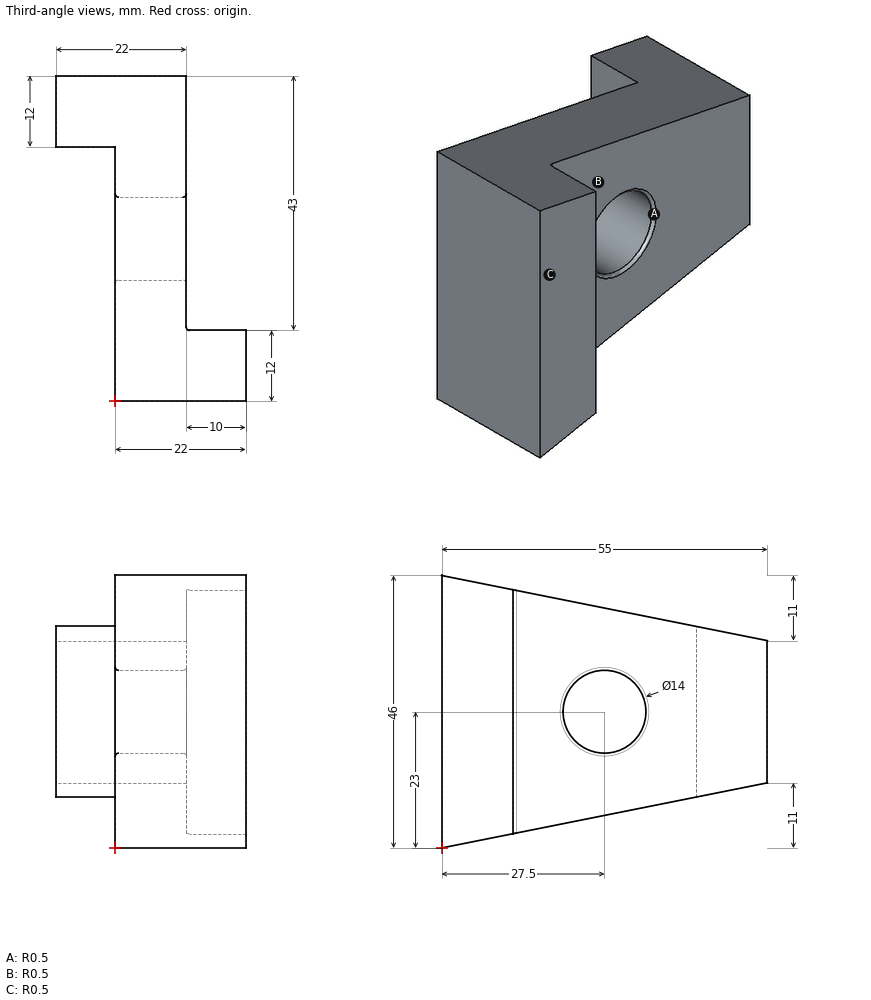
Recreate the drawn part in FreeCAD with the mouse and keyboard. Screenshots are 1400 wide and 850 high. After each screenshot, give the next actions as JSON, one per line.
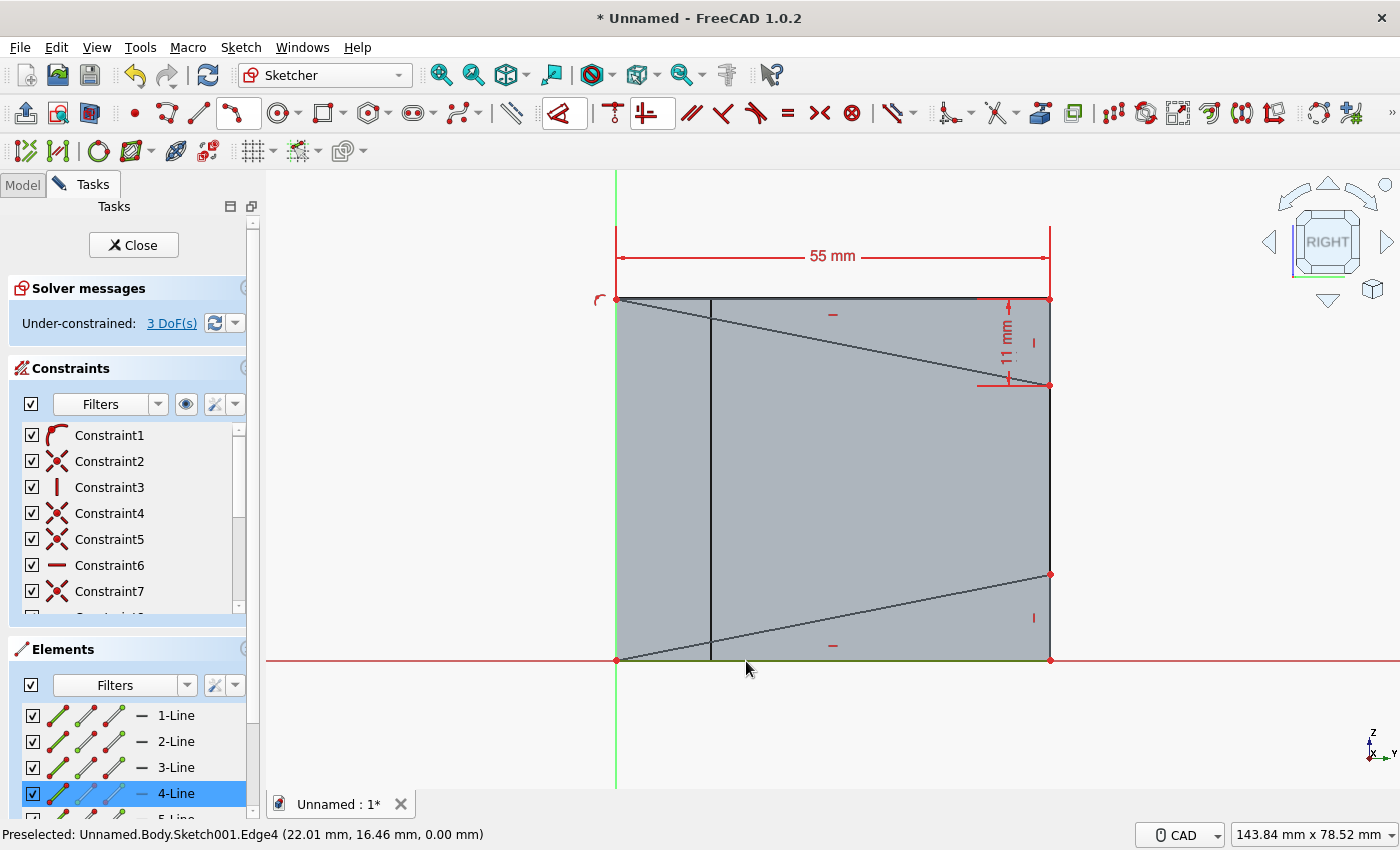
{"action": "key", "text": "l"}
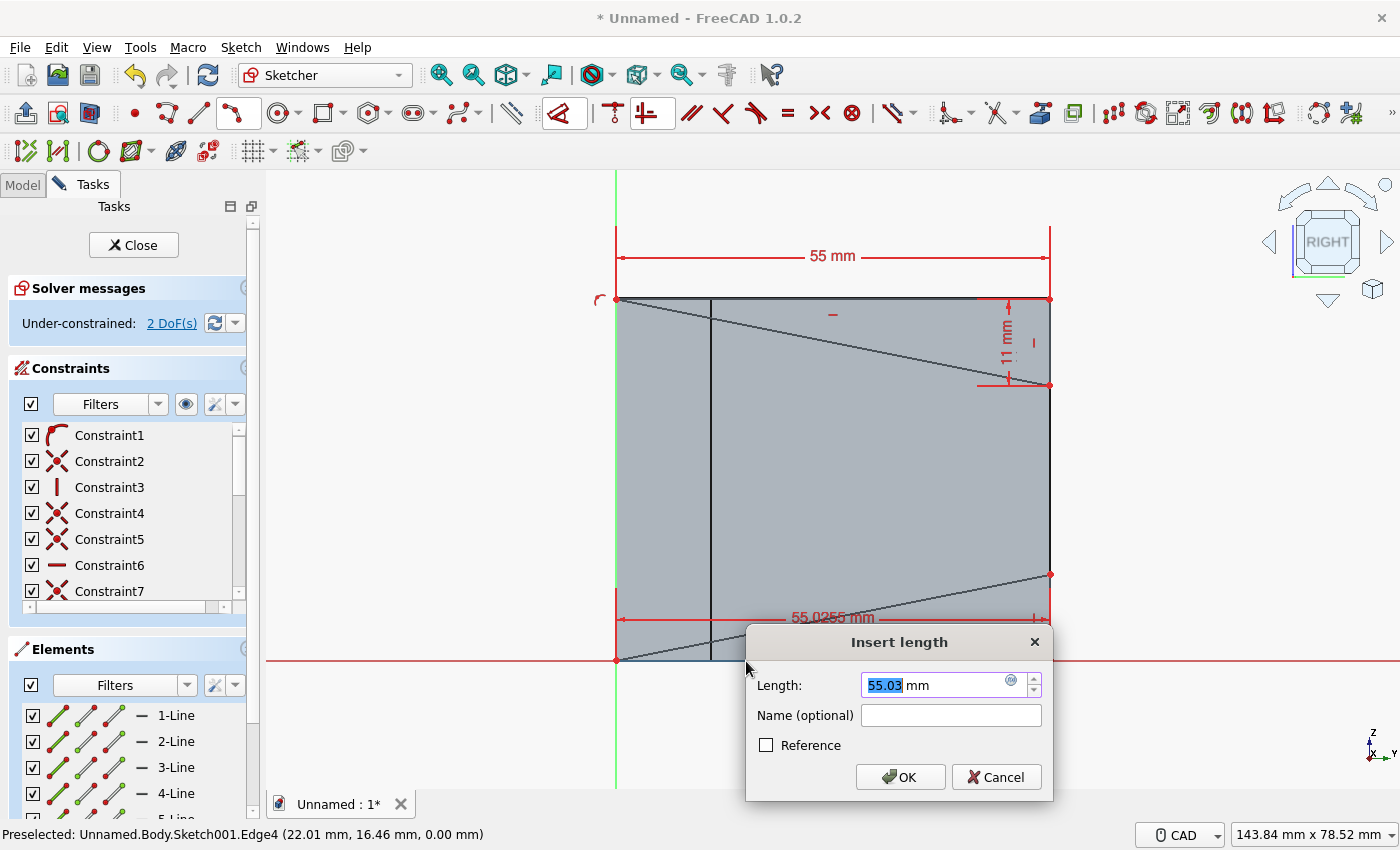
{"action": "type", "text": "55"}
{"action": "key", "text": "Return"}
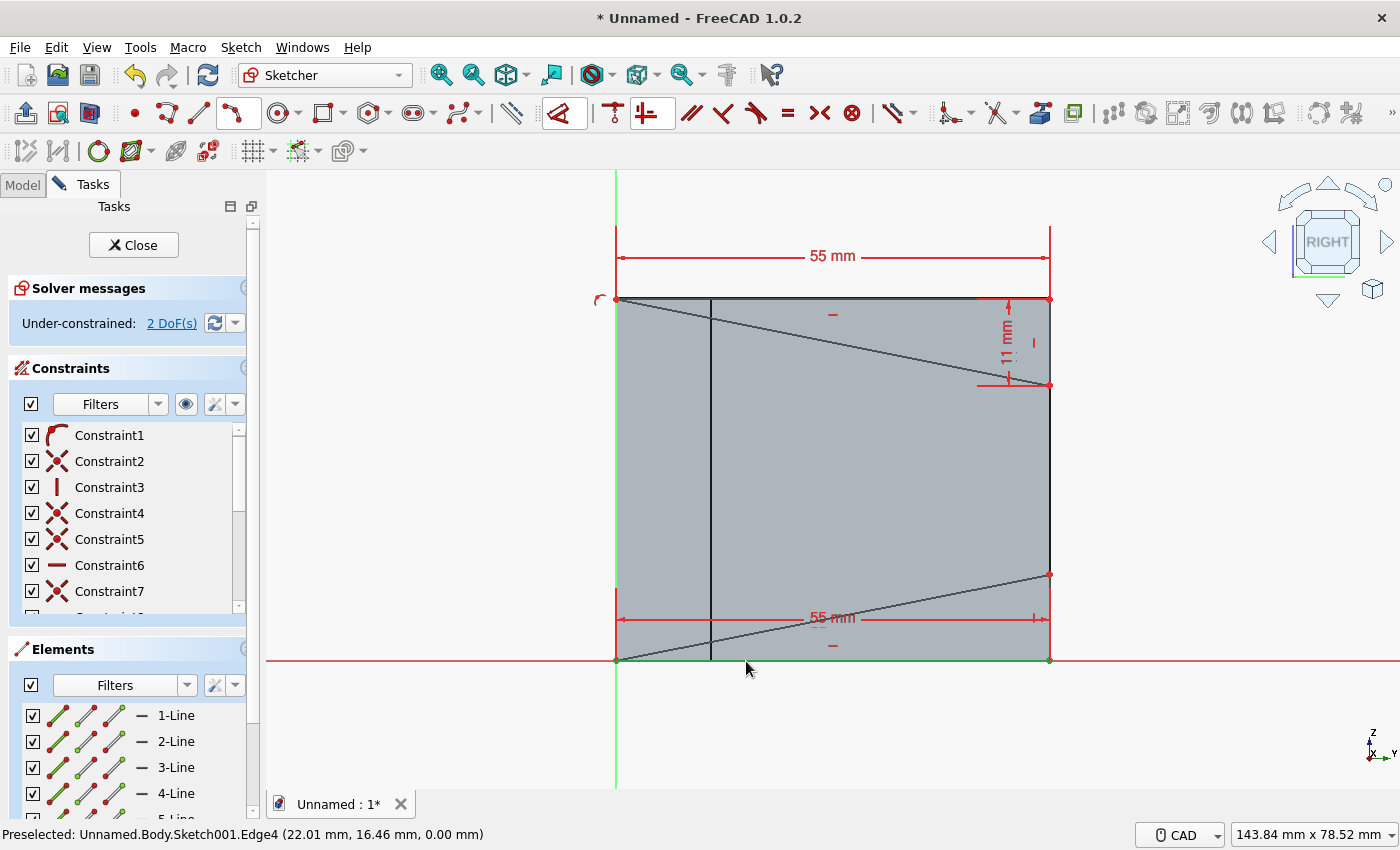
{"action": "left_click", "coordinate": [1050, 635]}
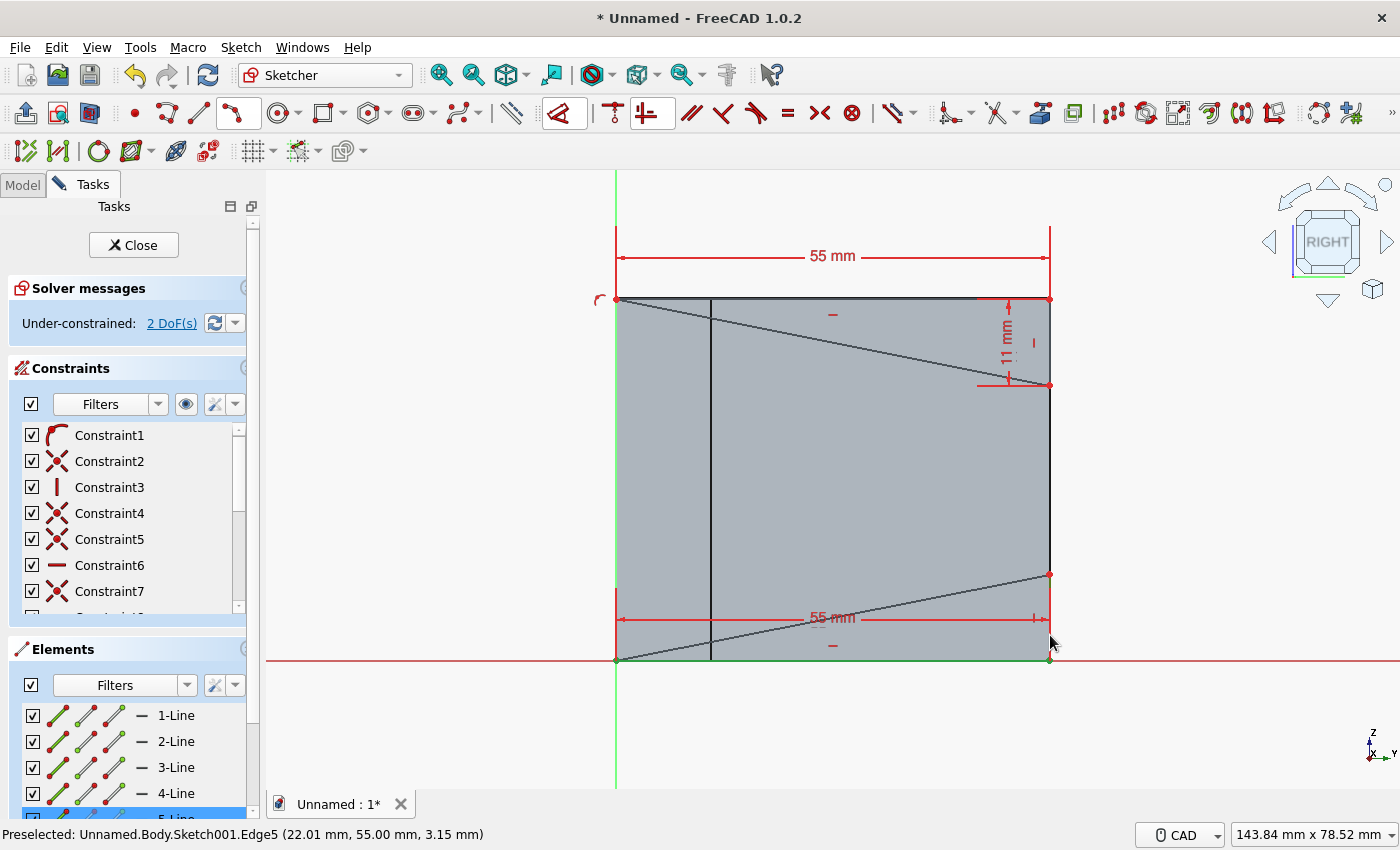
{"action": "key", "text": "i"}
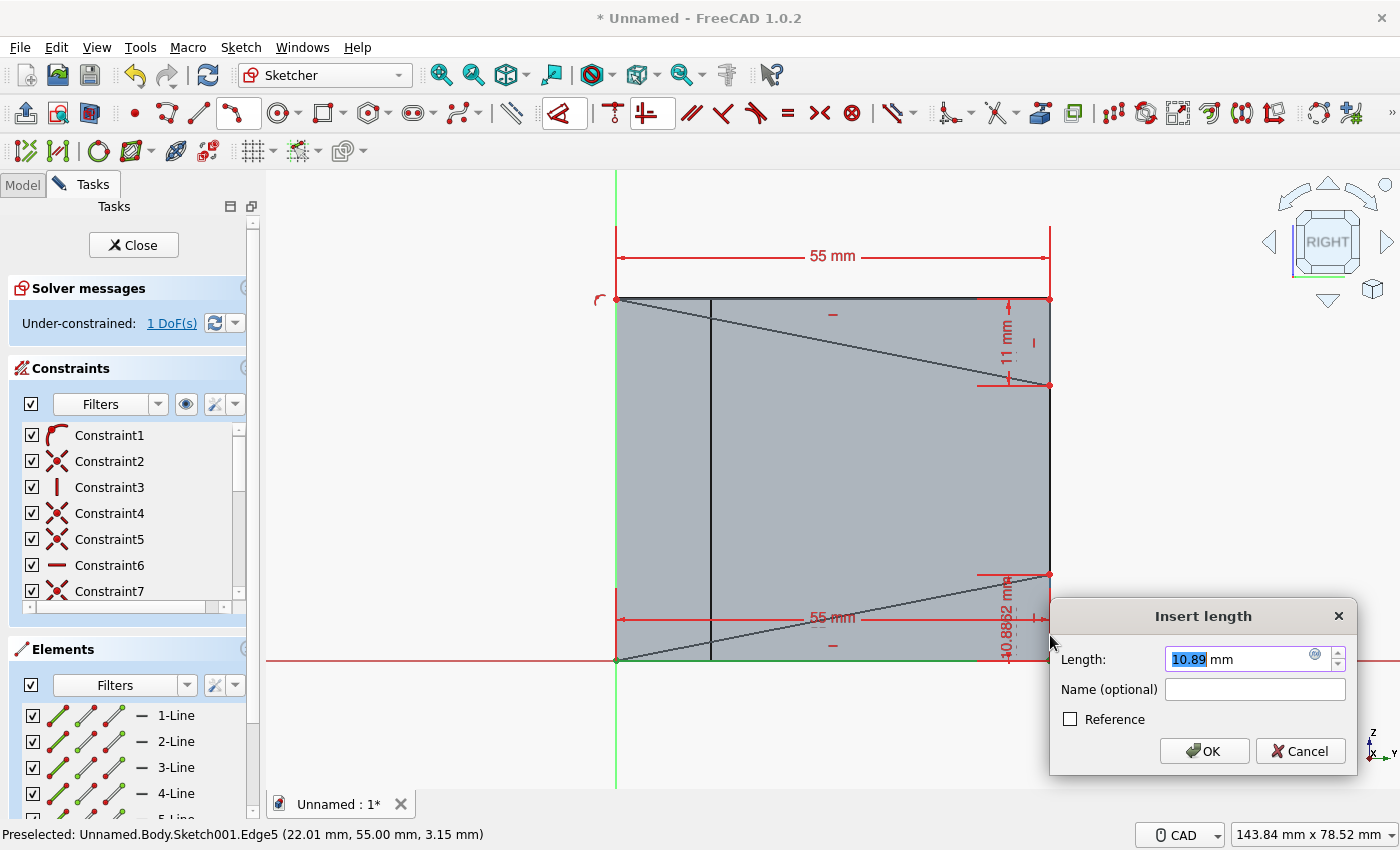
{"action": "type", "text": "11"}
{"action": "key", "text": "Return"}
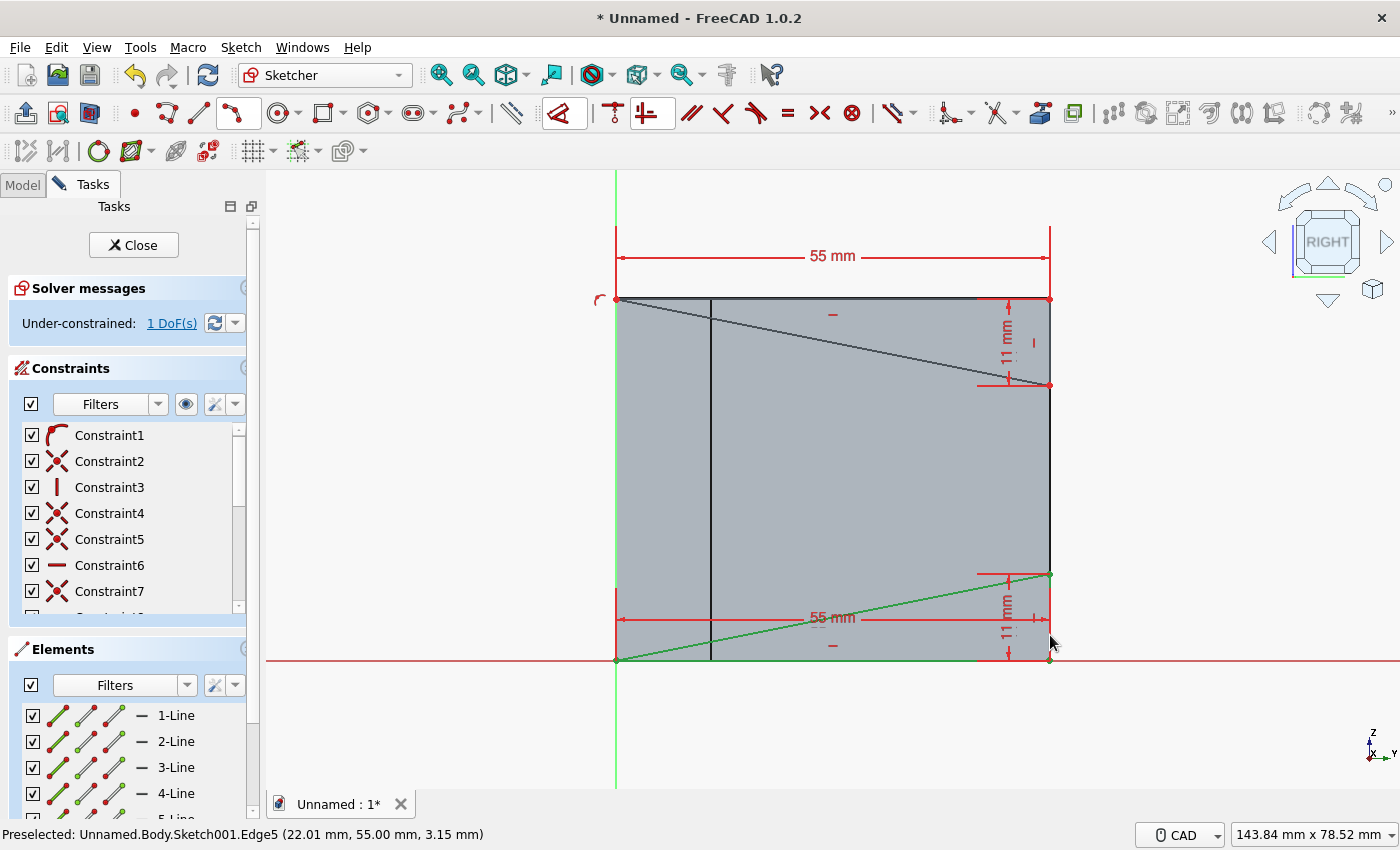
{"action": "left_click", "coordinate": [616, 299]}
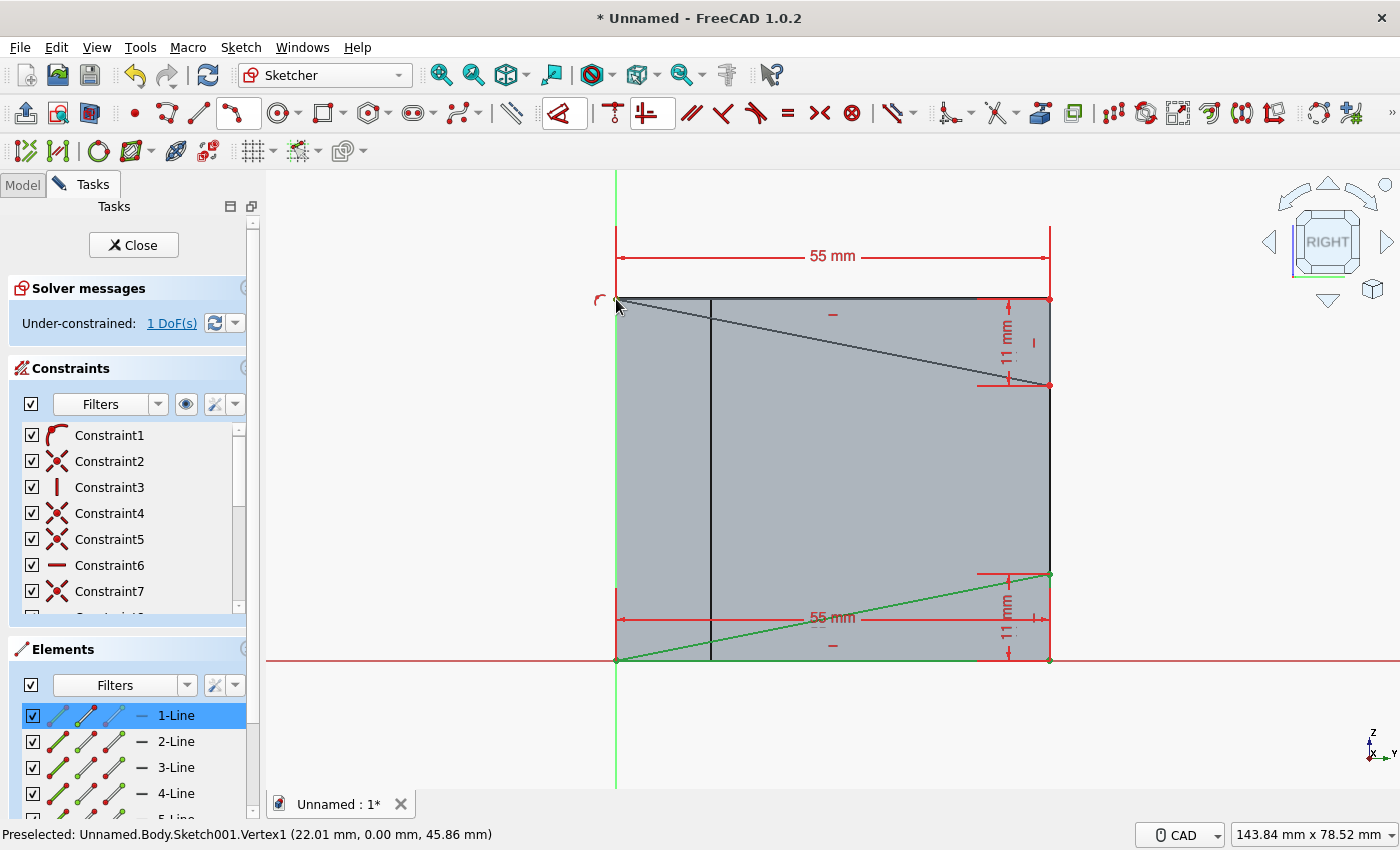
{"action": "left_click", "coordinate": [582, 114]}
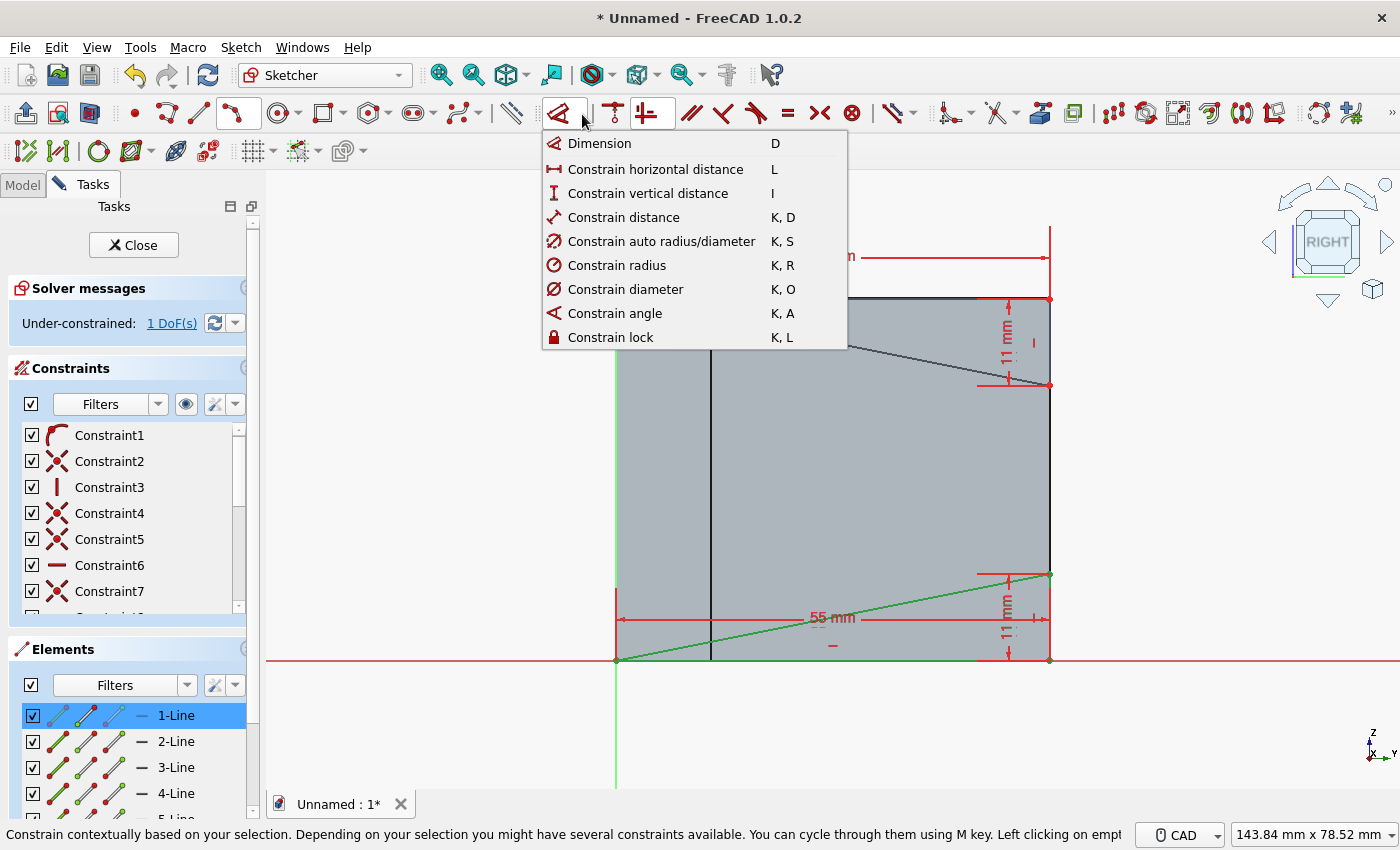
{"action": "left_click", "coordinate": [695, 193]}